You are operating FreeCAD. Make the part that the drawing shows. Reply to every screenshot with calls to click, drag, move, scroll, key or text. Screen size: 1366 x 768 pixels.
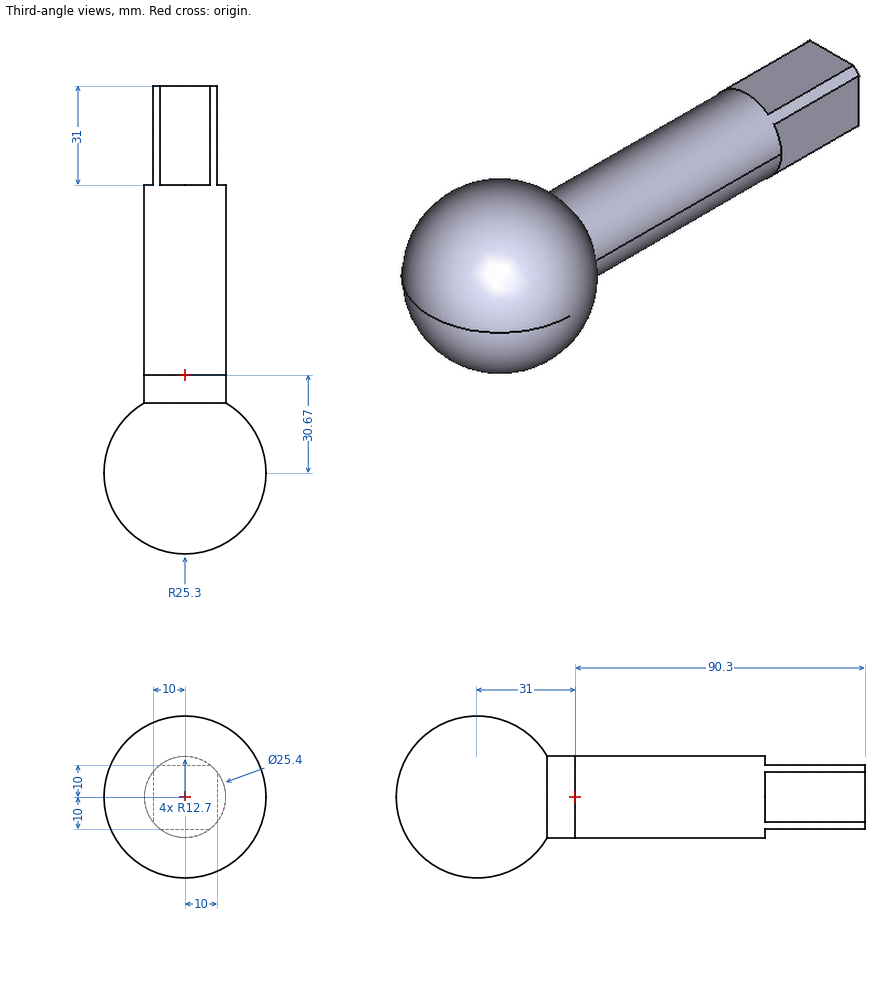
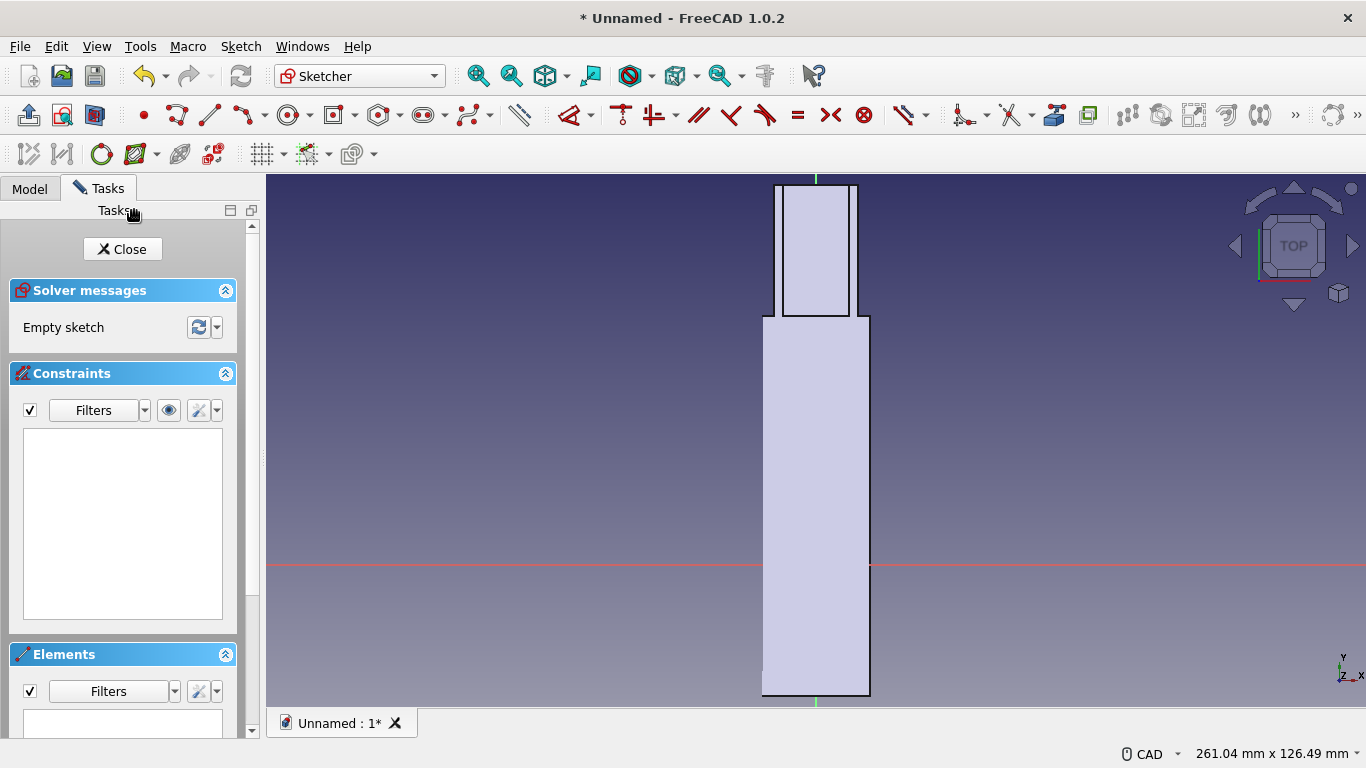
scroll(748, 440, down, 5)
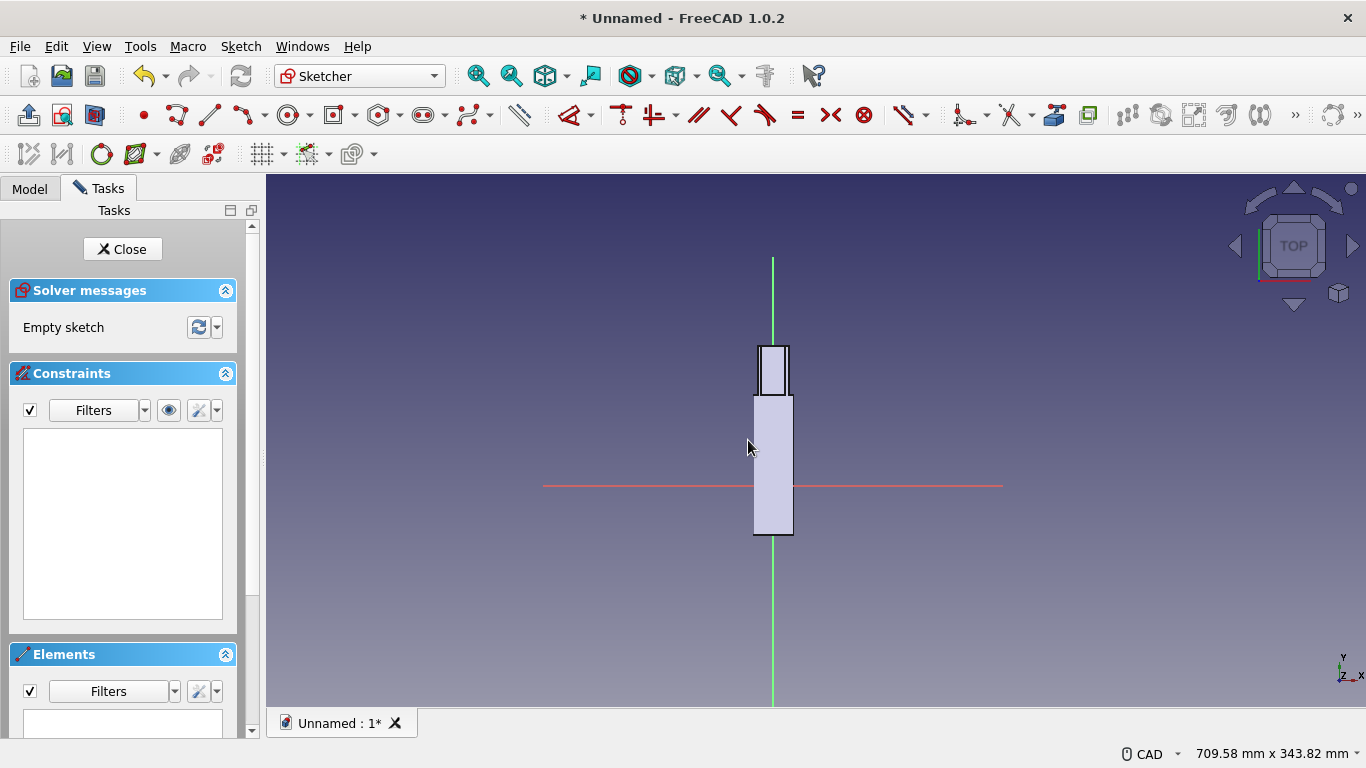
scroll(803, 559, up, 7)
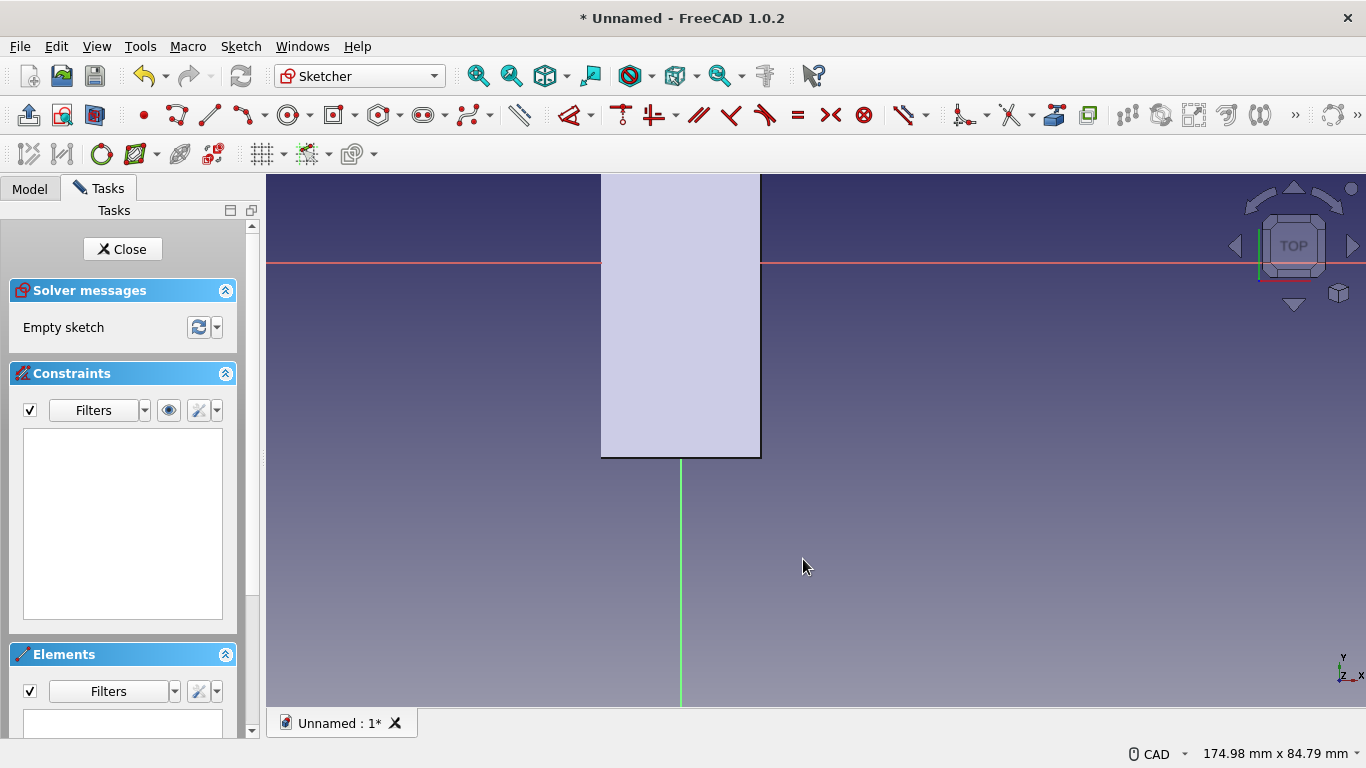
click(210, 116)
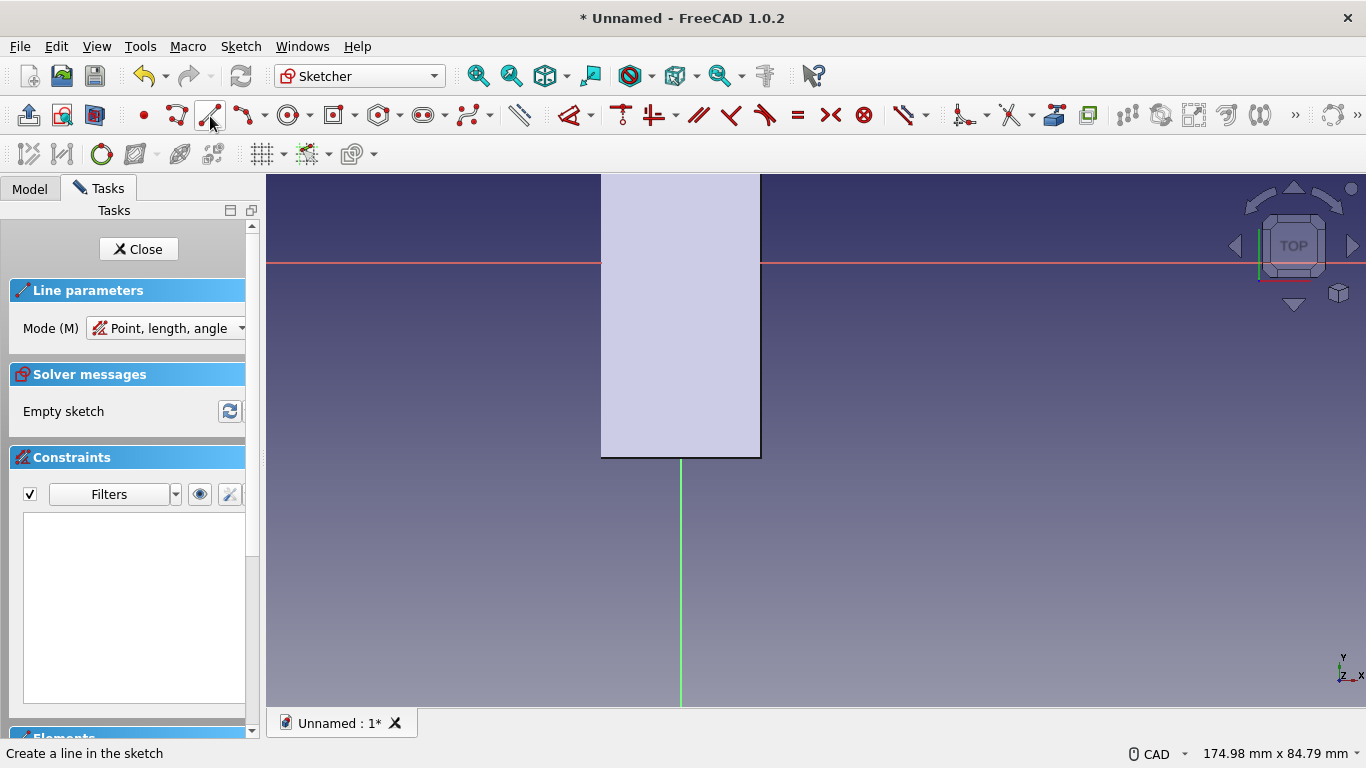
click(840, 455)
click(522, 455)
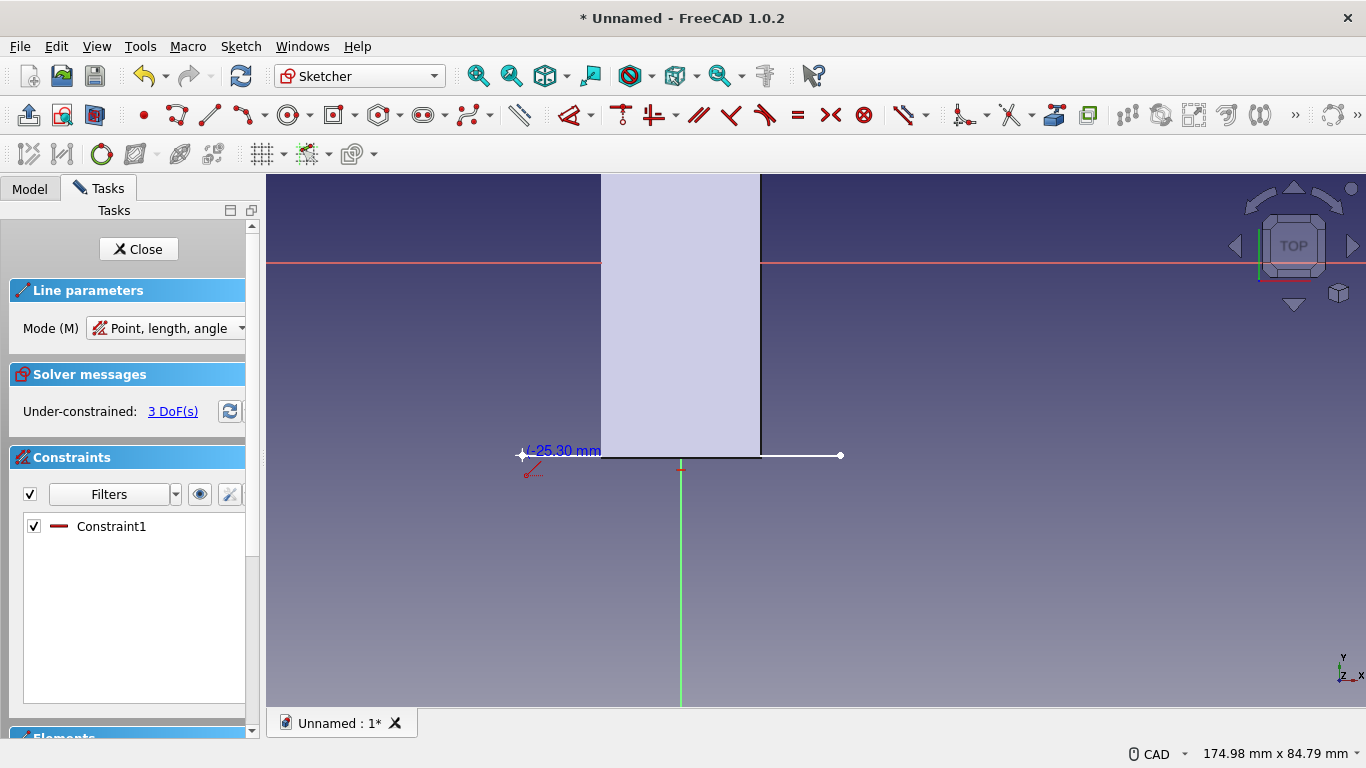
click(242, 116)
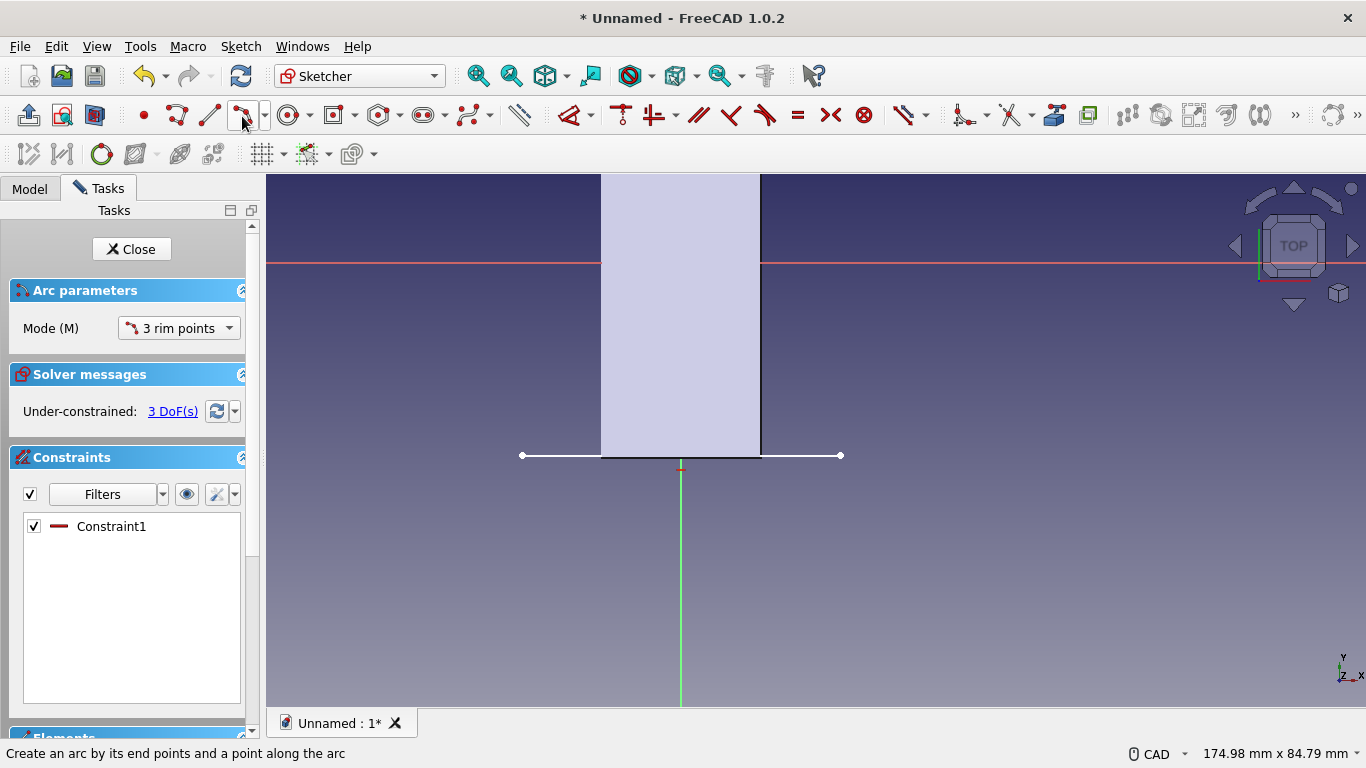
click(522, 456)
click(840, 456)
click(632, 607)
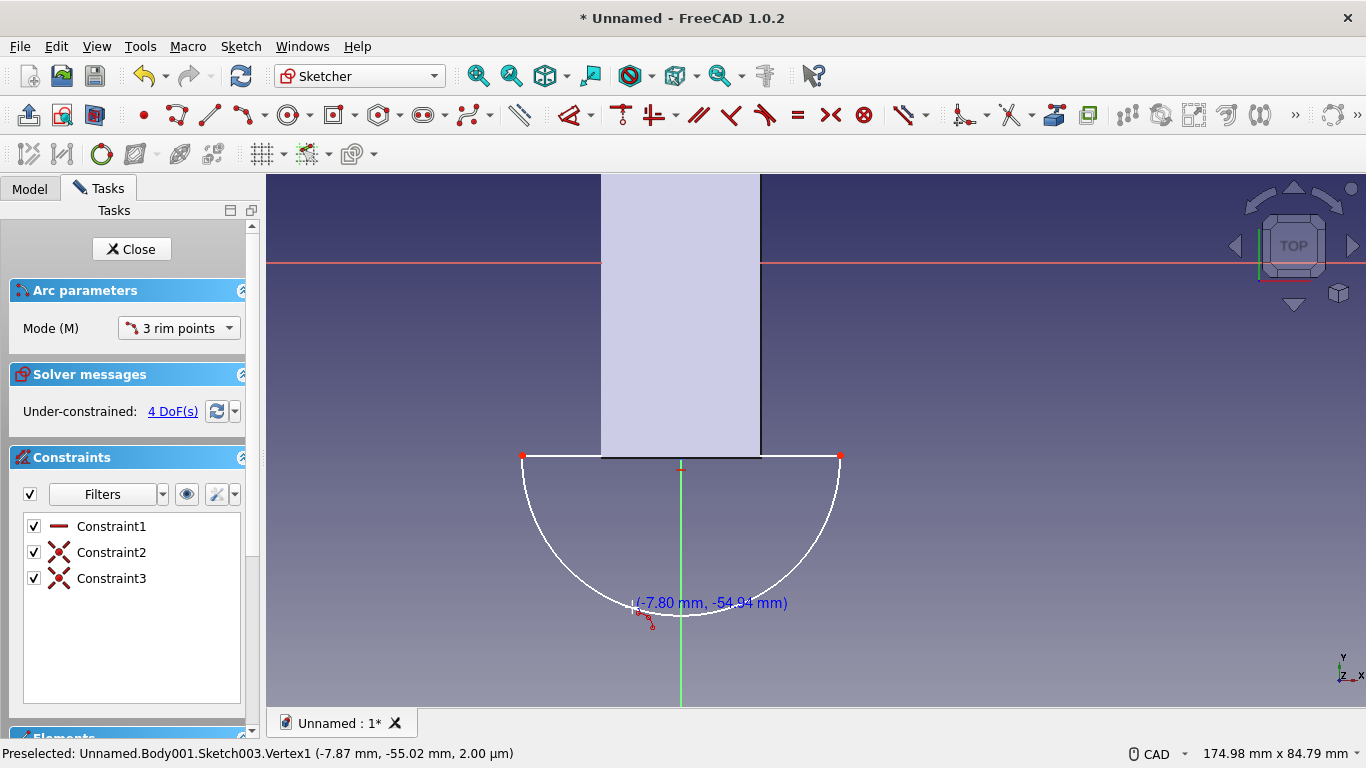
click(210, 116)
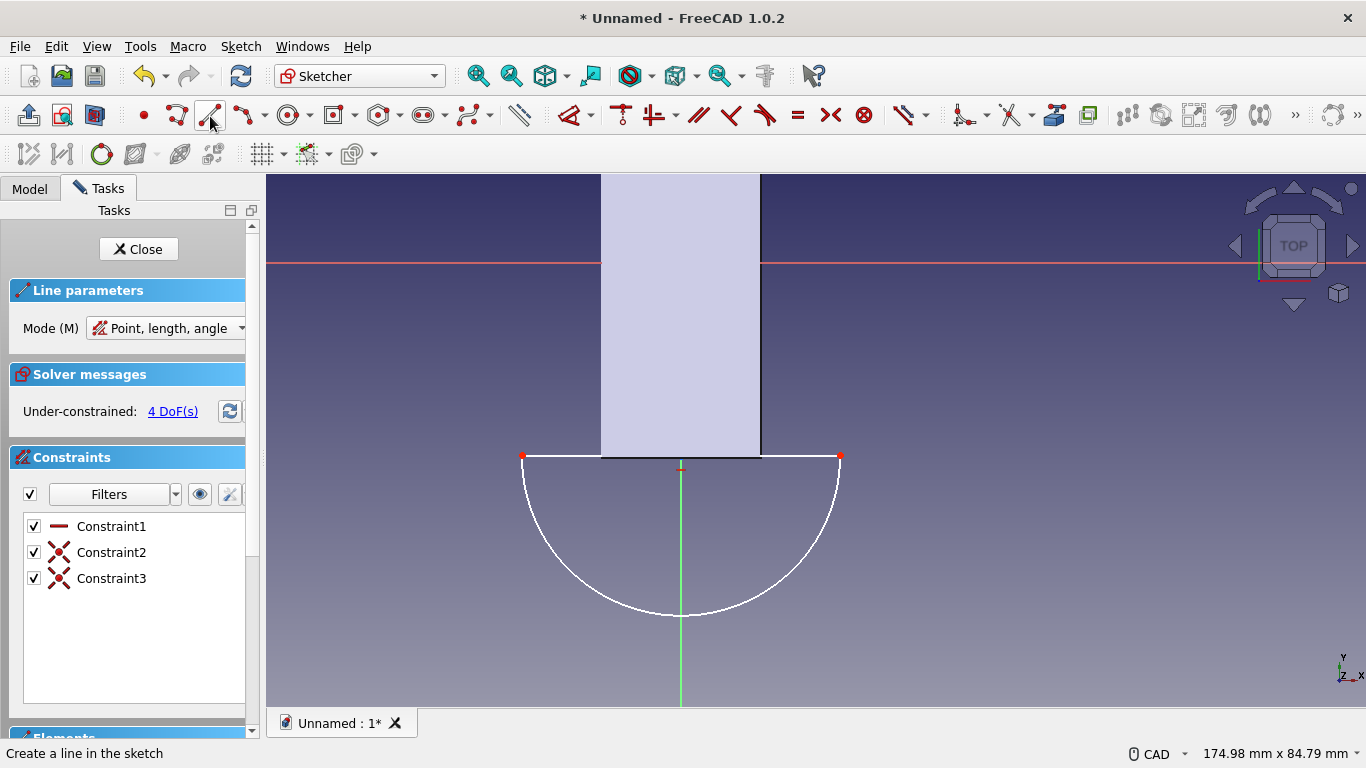
click(872, 455)
click(967, 455)
key(Escape)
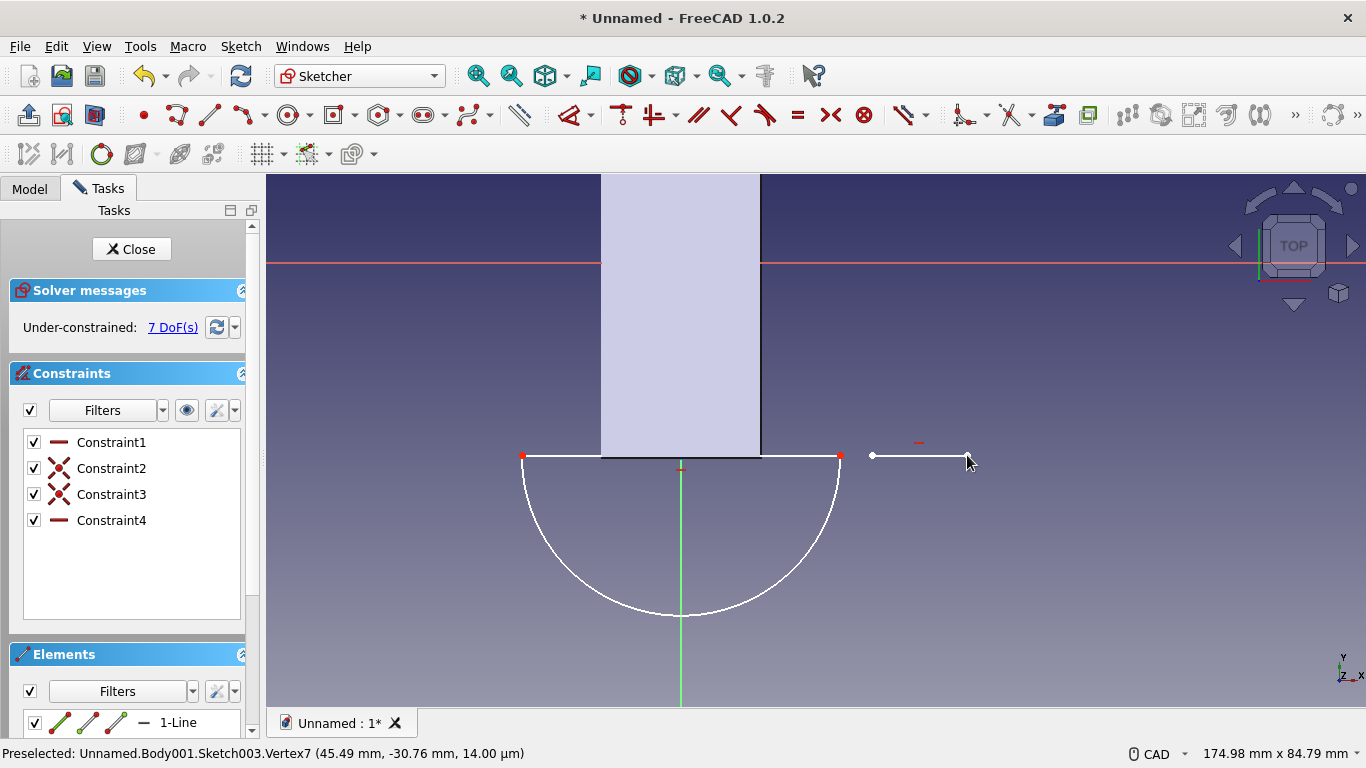
click(901, 456)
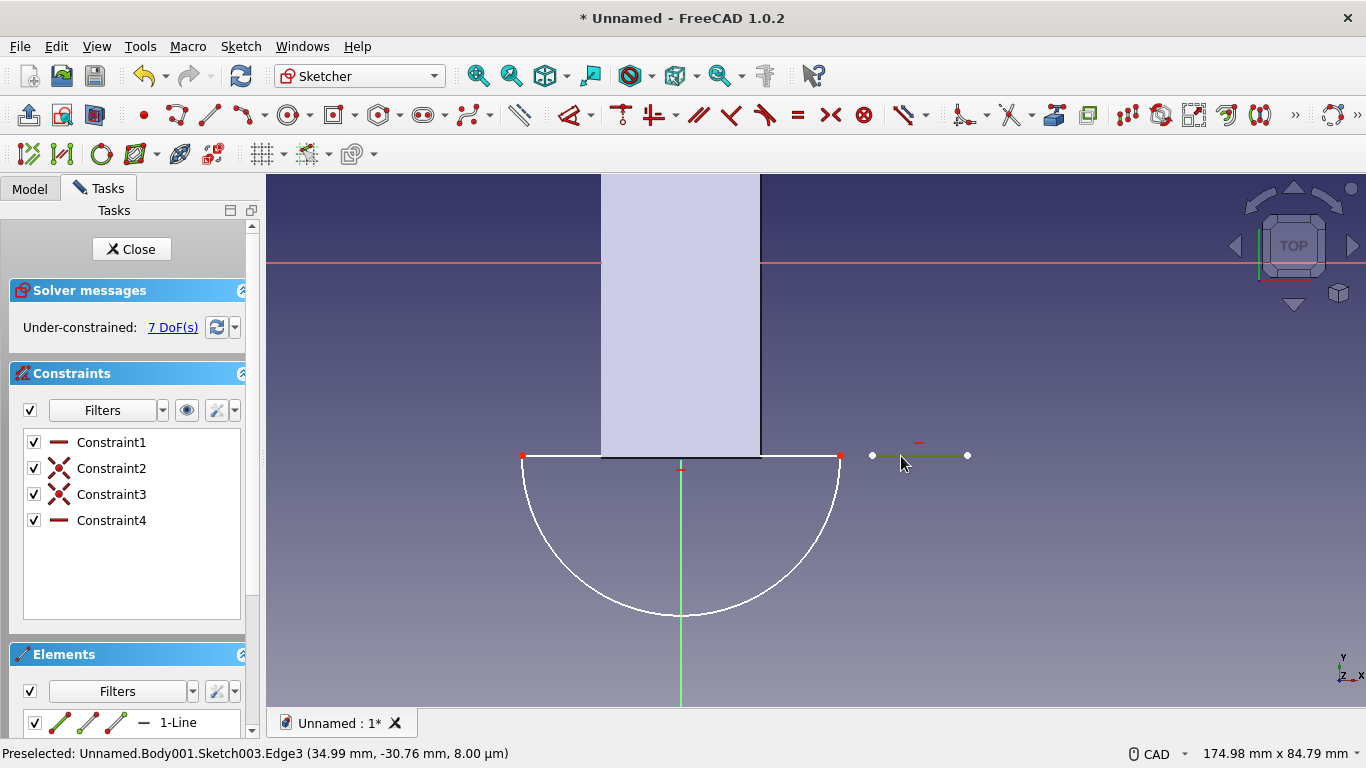
key(g)
key(n)